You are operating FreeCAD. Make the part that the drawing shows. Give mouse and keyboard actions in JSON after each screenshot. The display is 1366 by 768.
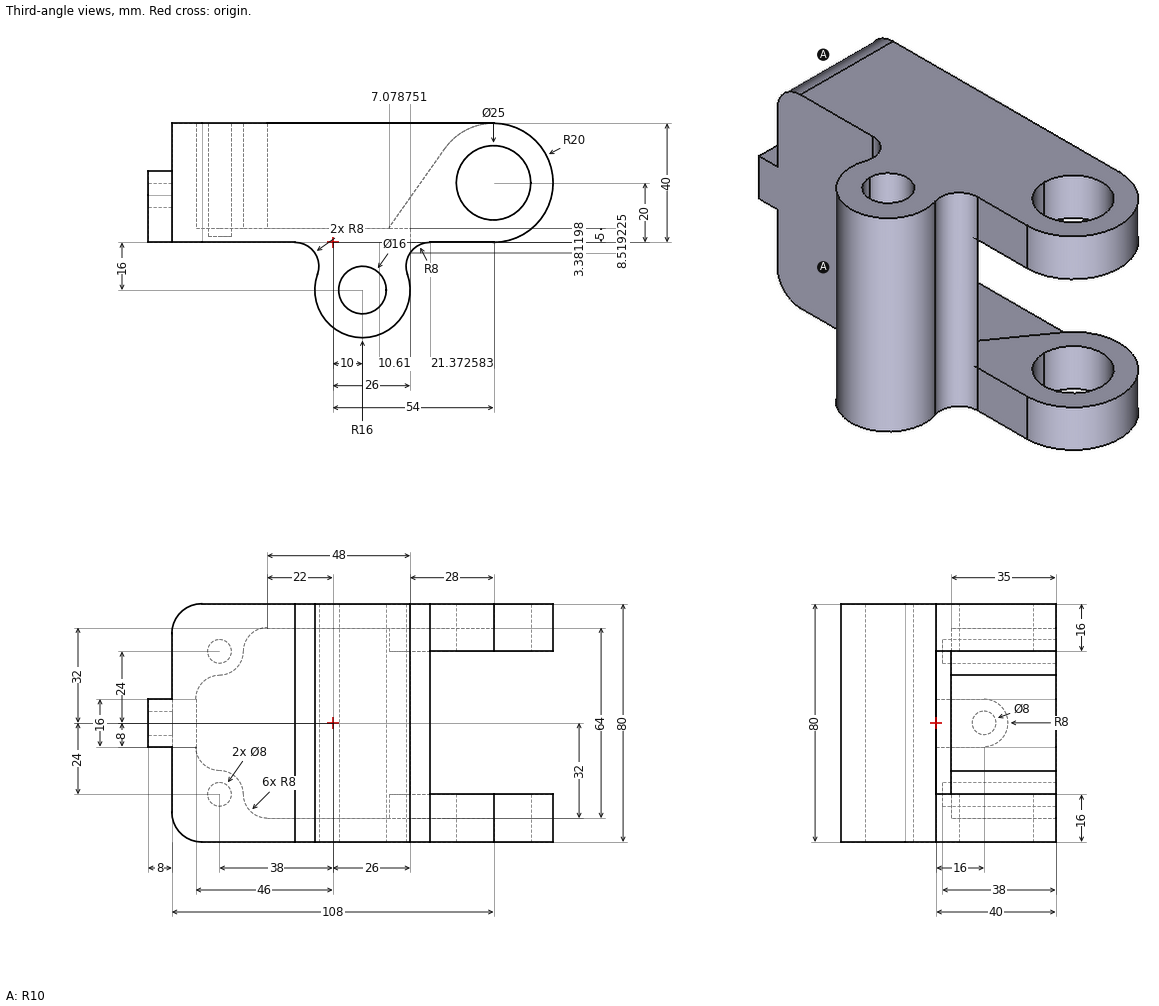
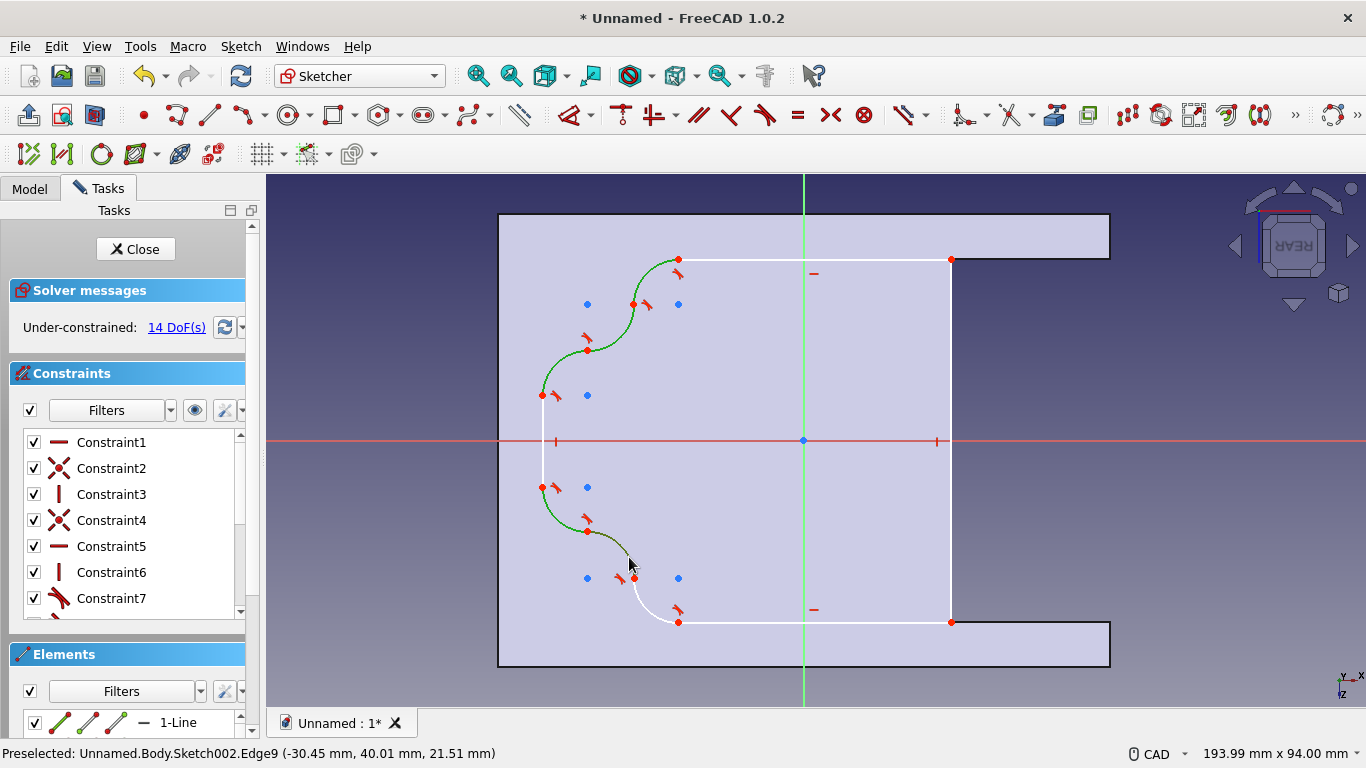
{"action": "left_click", "coordinate": [639, 598]}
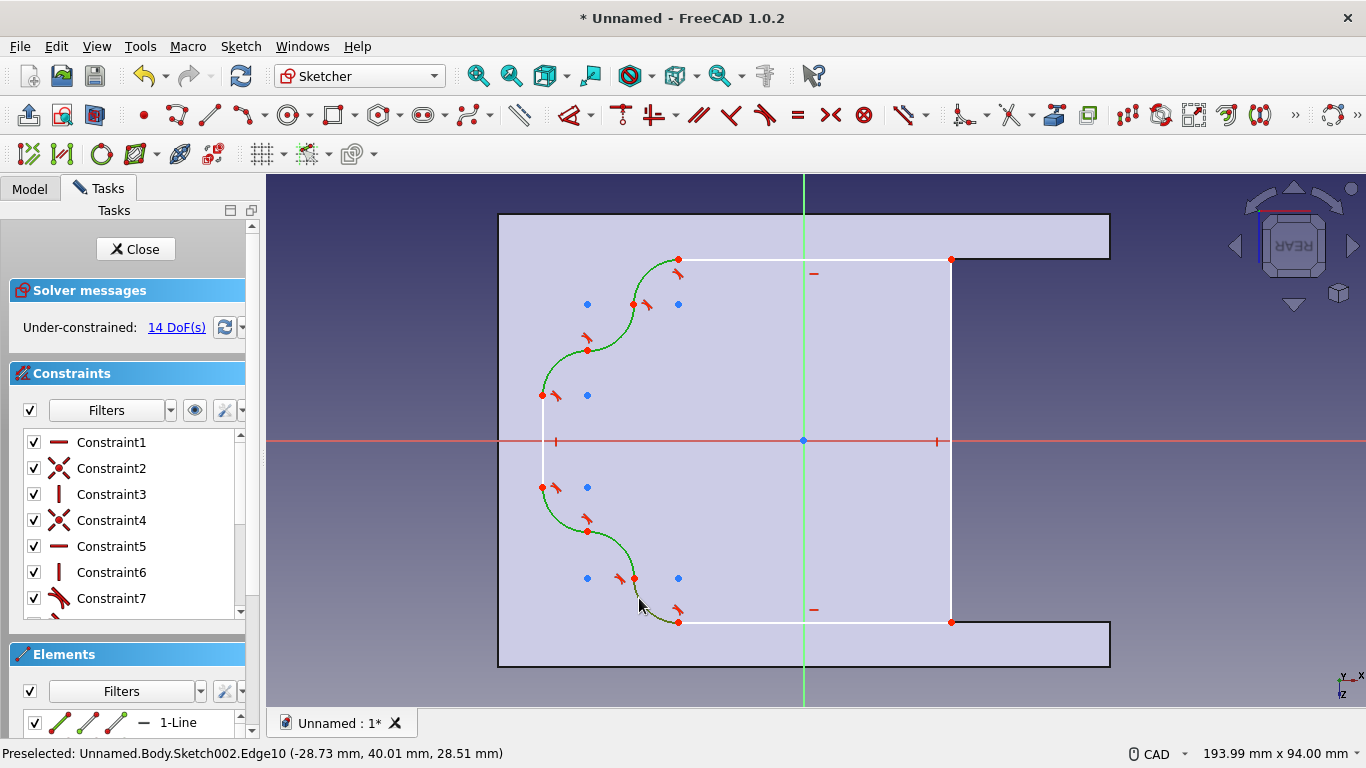
{"action": "left_click", "coordinate": [798, 116]}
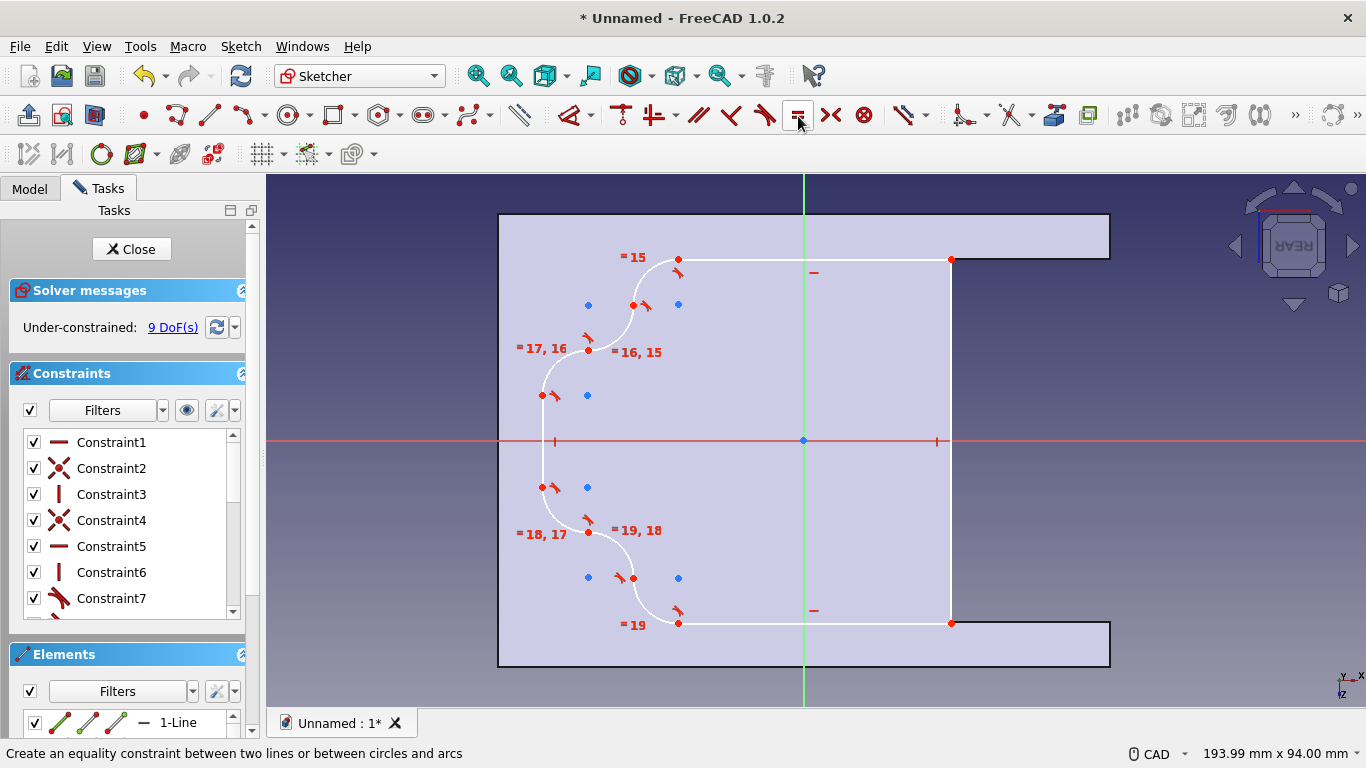
{"action": "left_click", "coordinate": [568, 116]}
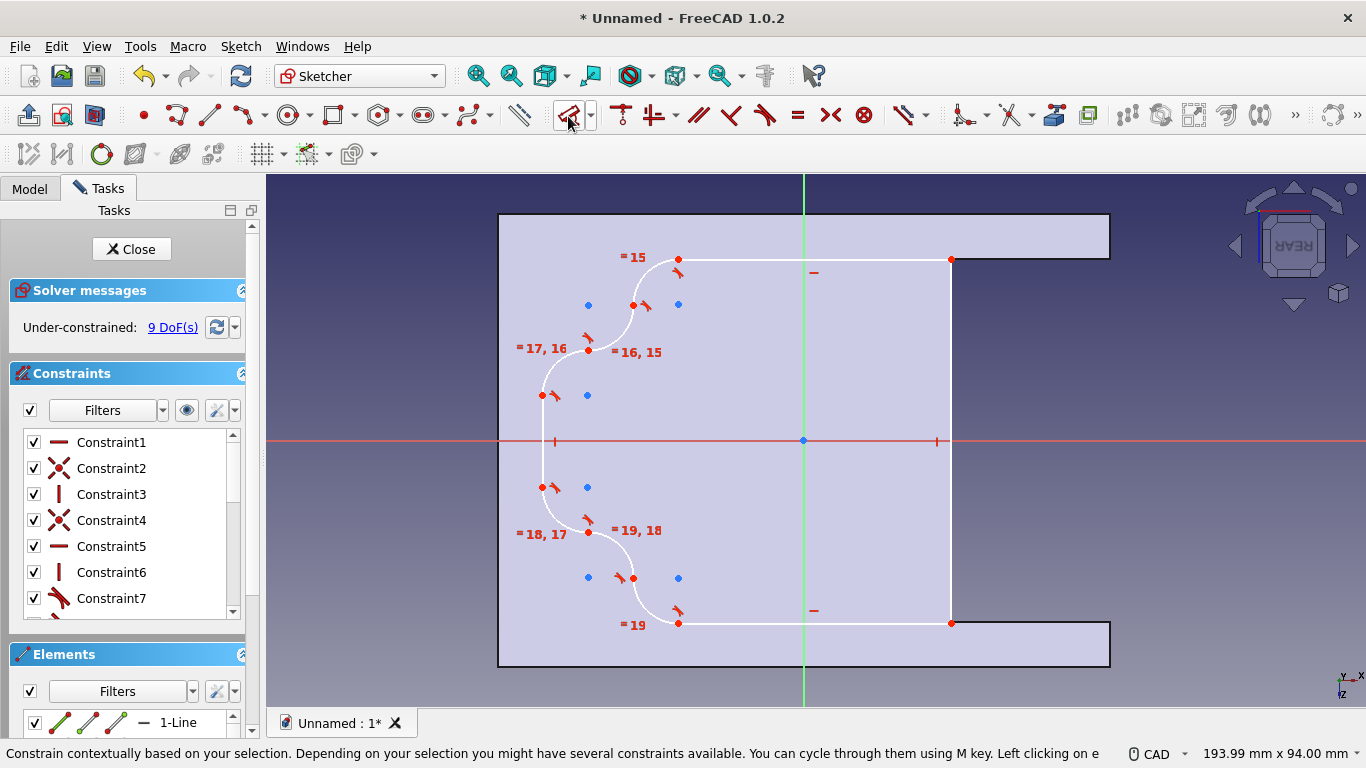
{"action": "left_click", "coordinate": [658, 265]}
{"action": "left_click", "coordinate": [643, 237]}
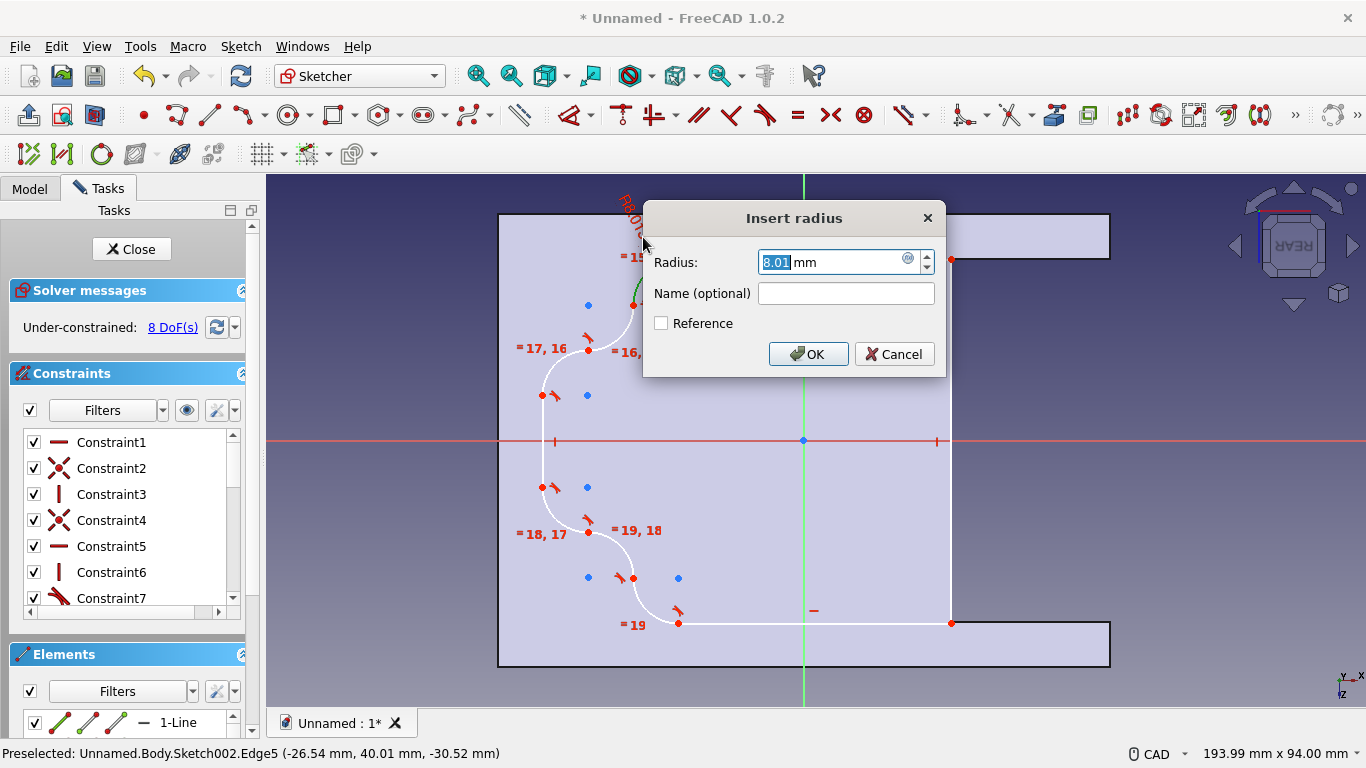
{"action": "type", "text": "8"}
{"action": "key", "text": "Return"}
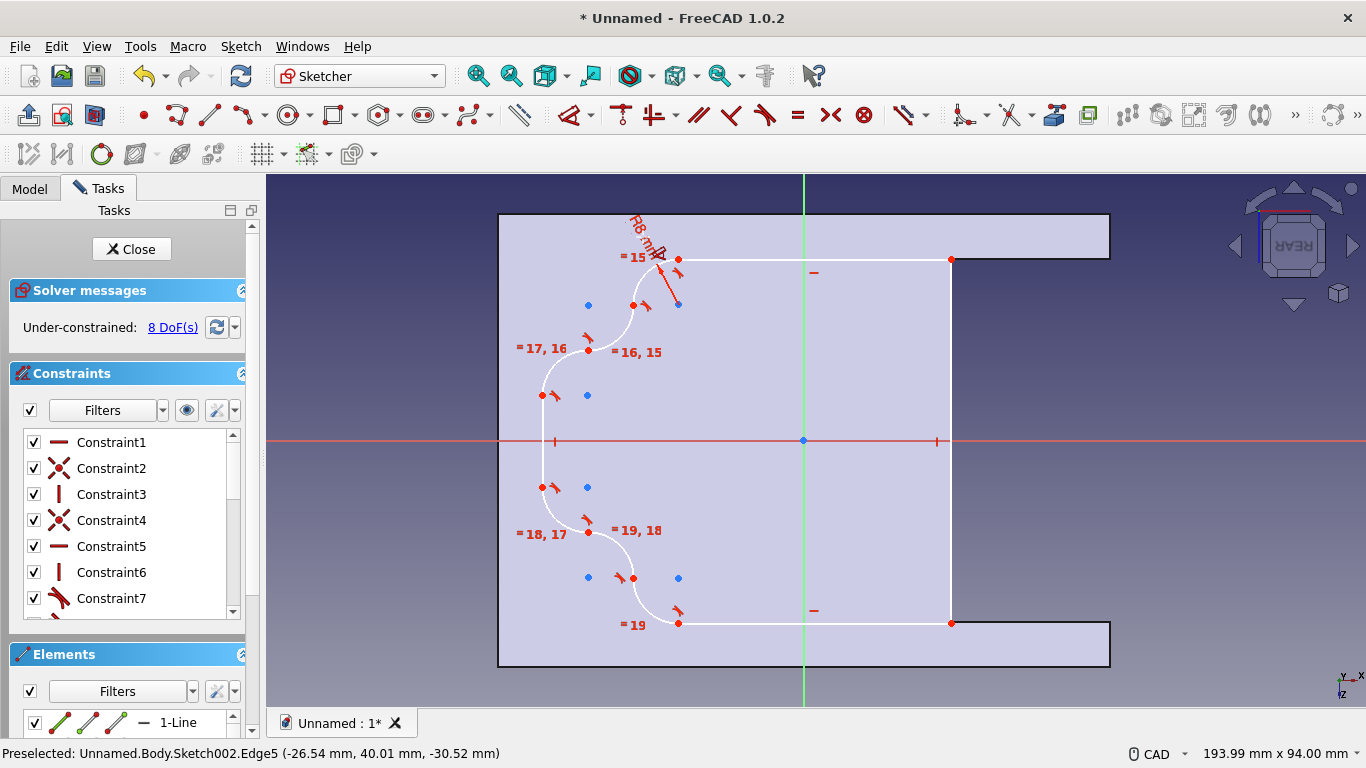
{"action": "left_click", "coordinate": [760, 624]}
{"action": "left_click", "coordinate": [752, 658]}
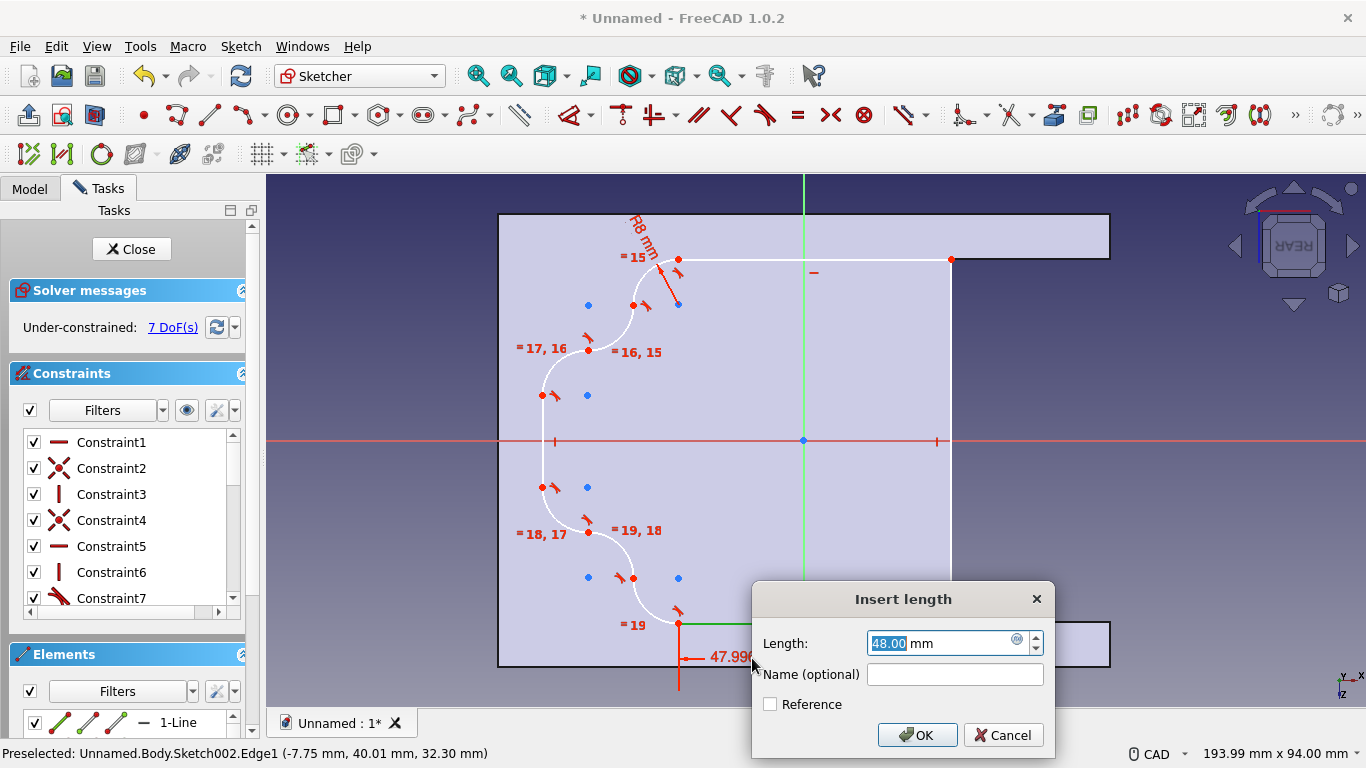
{"action": "type", "text": "48"}
{"action": "key", "text": "Return"}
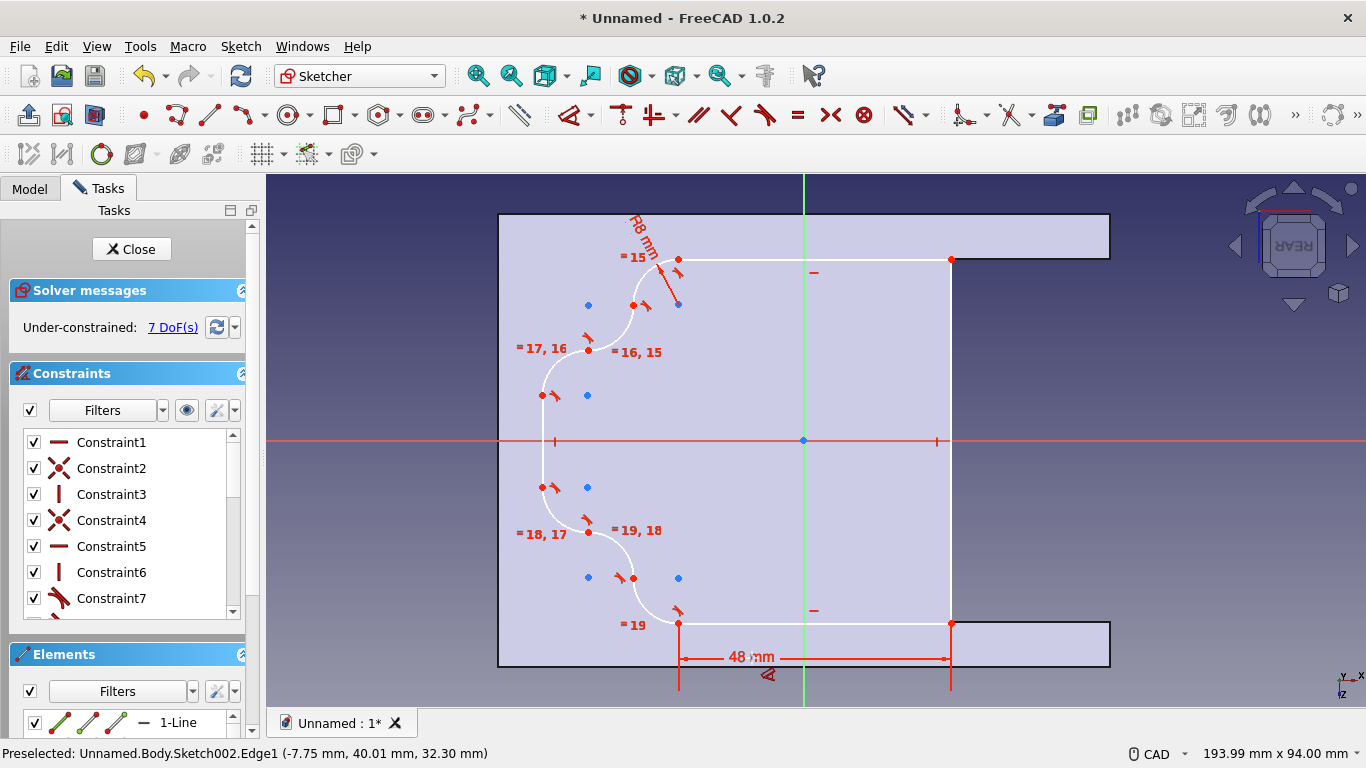
{"action": "left_click", "coordinate": [951, 514]}
{"action": "left_click", "coordinate": [985, 358]}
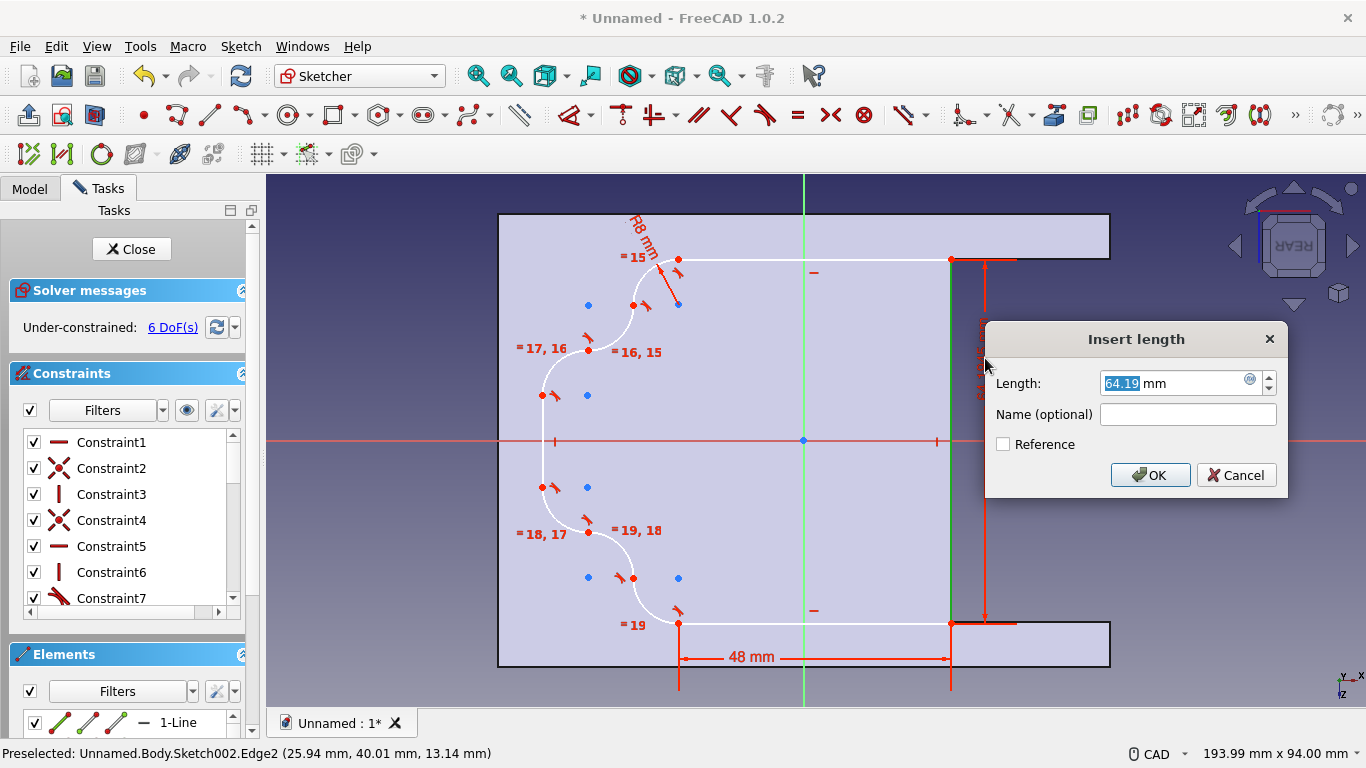
{"action": "type", "text": "64"}
{"action": "key", "text": "Return"}